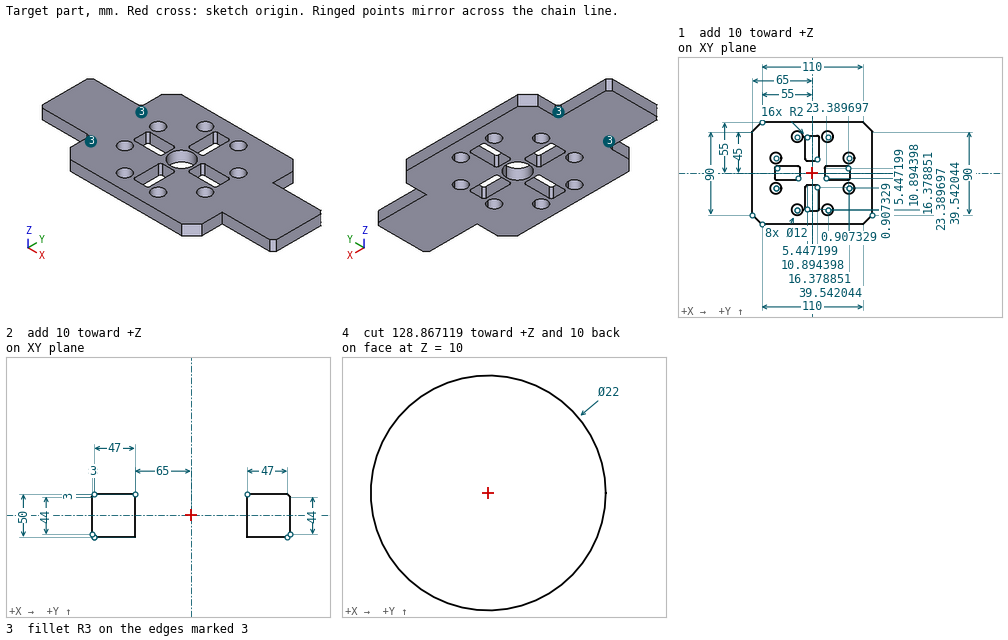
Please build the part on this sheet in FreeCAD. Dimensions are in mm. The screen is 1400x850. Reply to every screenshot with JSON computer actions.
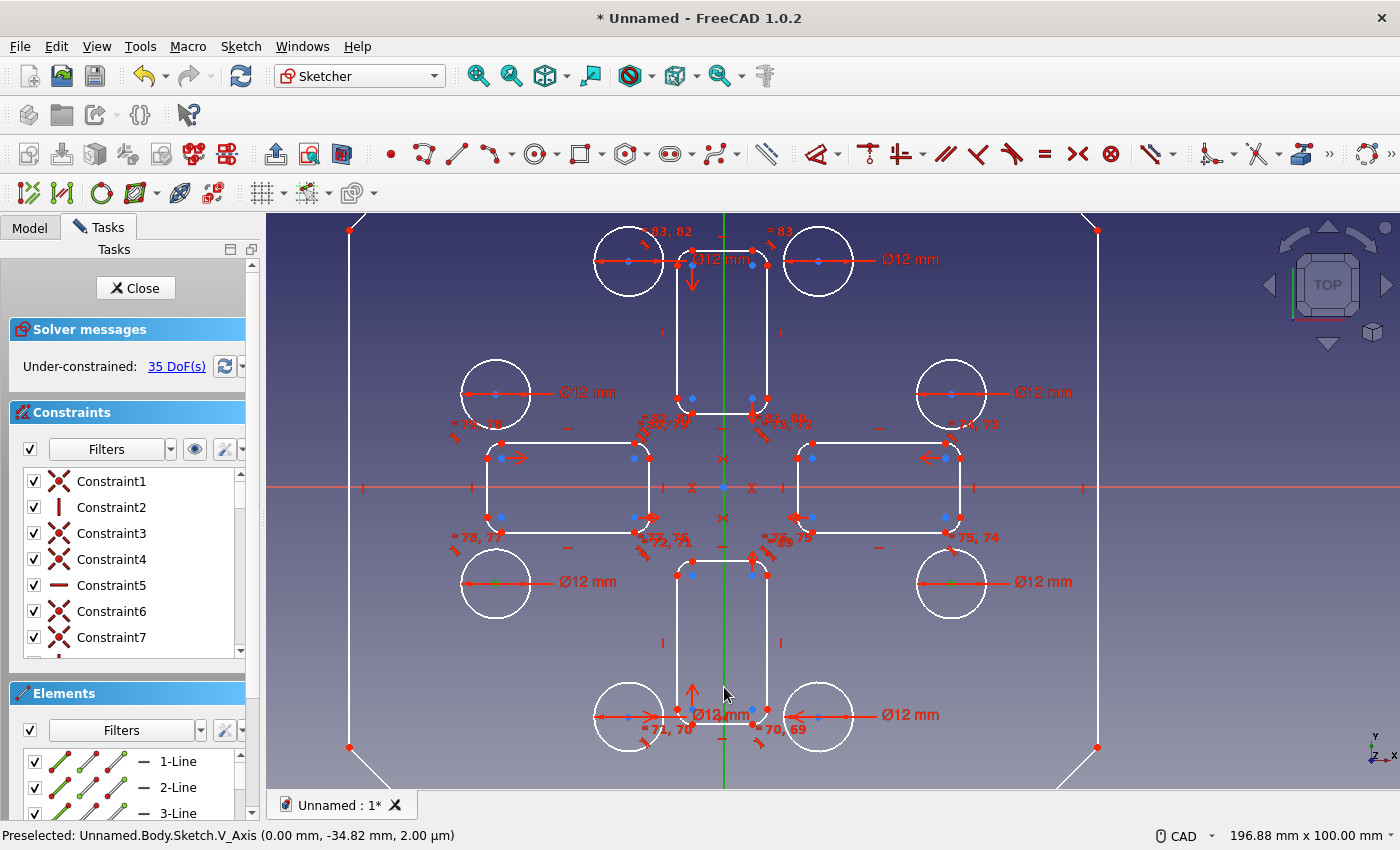
{"action": "left_click", "coordinate": [1078, 154]}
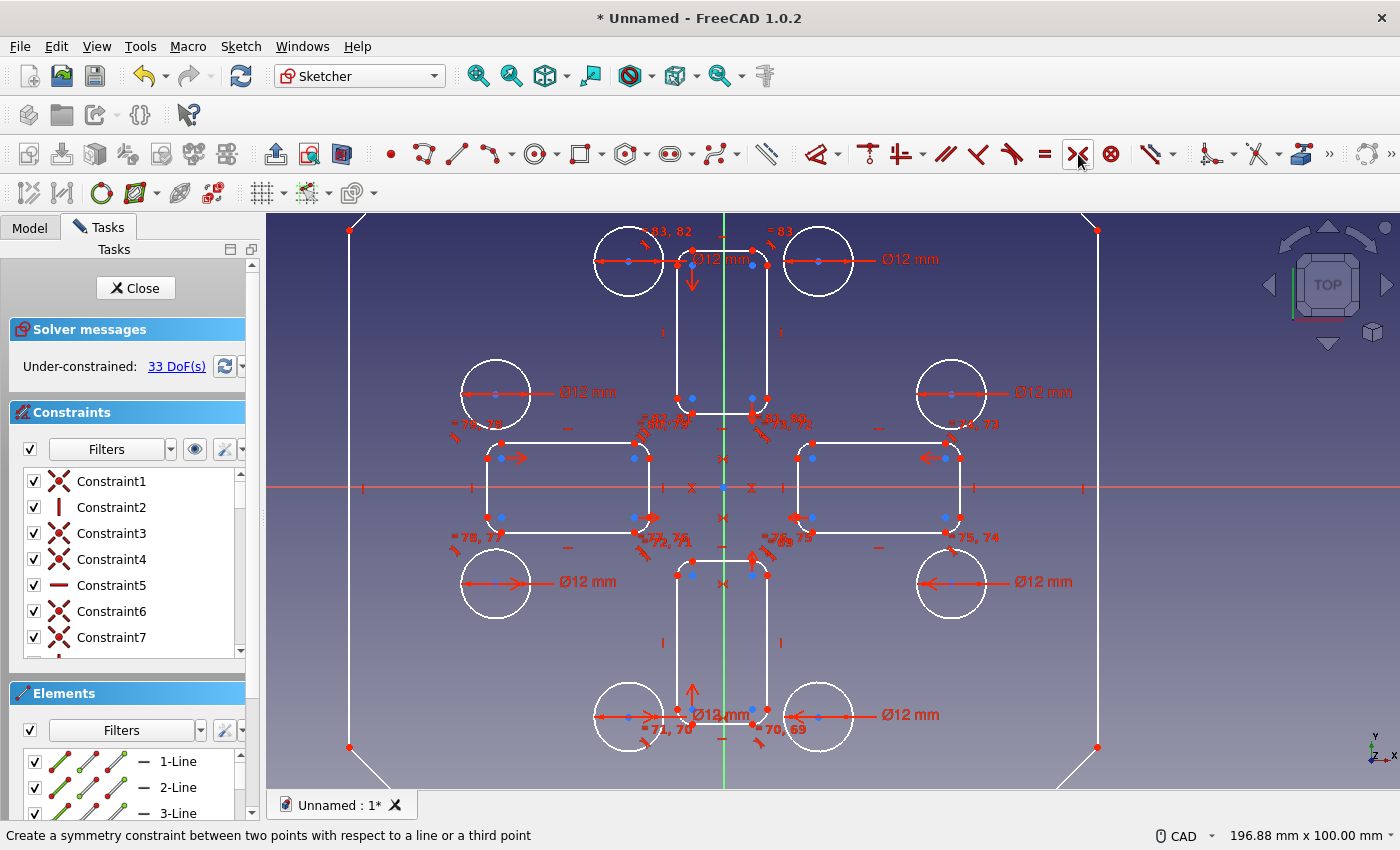
{"action": "left_click", "coordinate": [951, 584]}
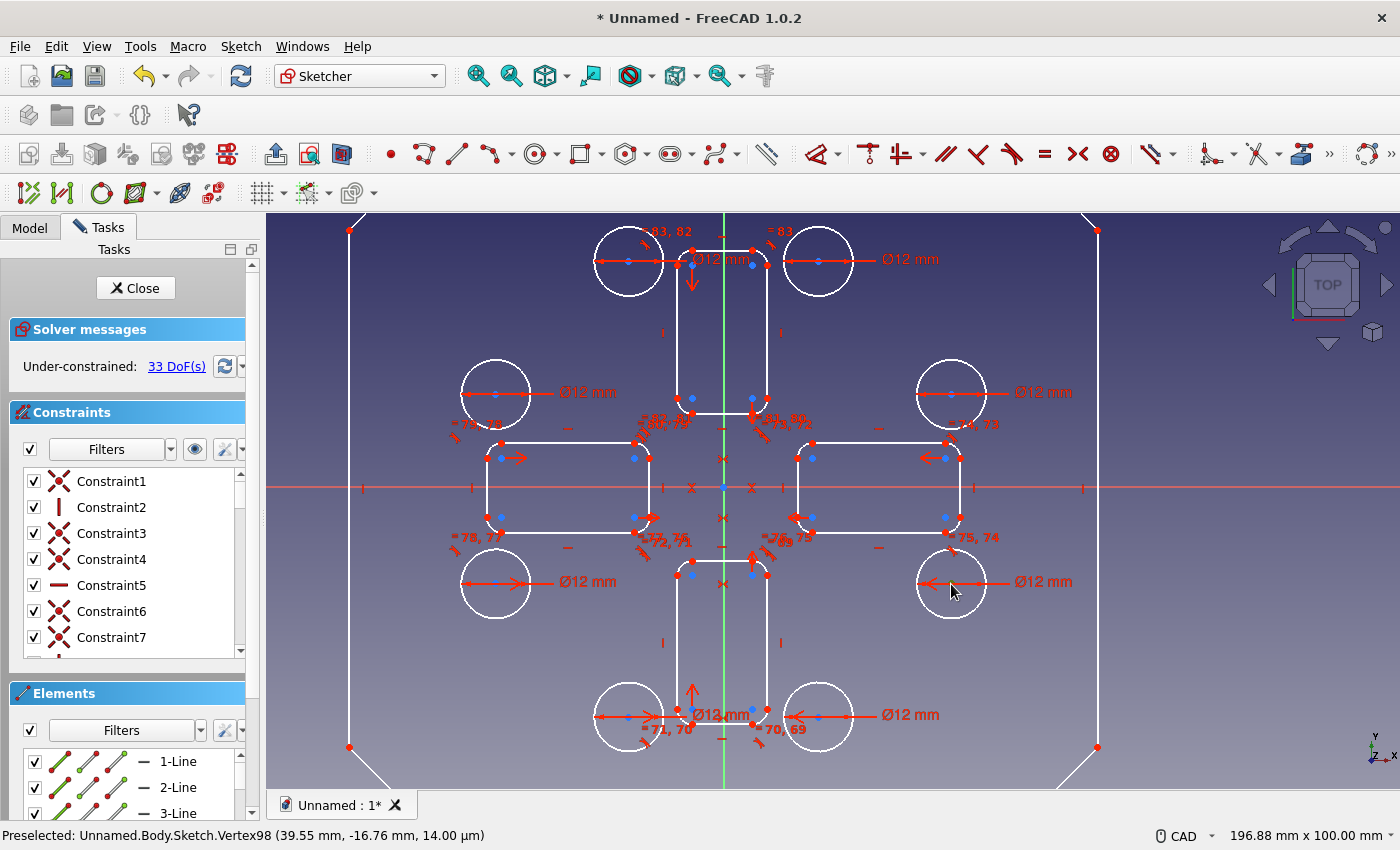
{"action": "left_click", "coordinate": [951, 394]}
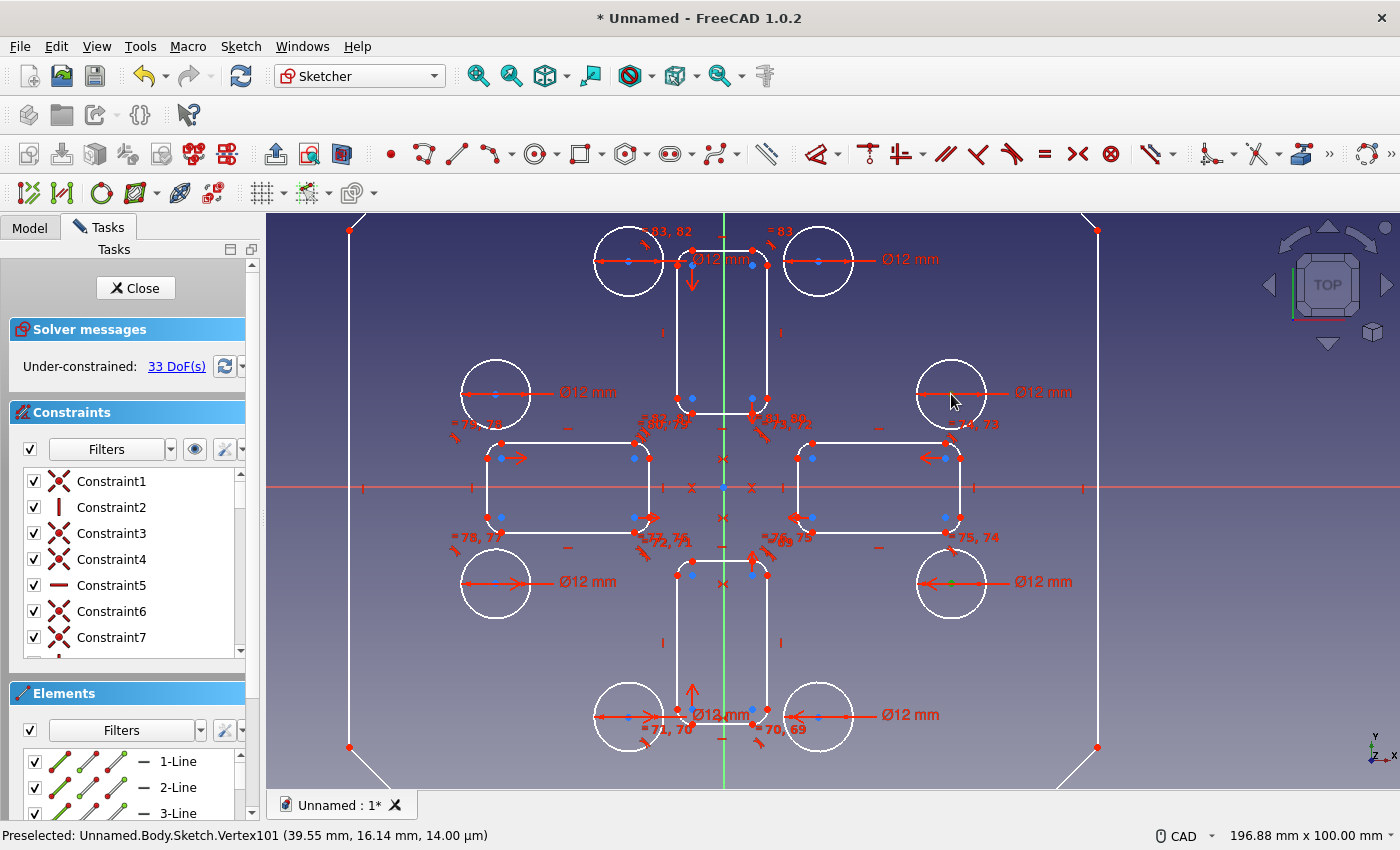
{"action": "left_click", "coordinate": [428, 487]}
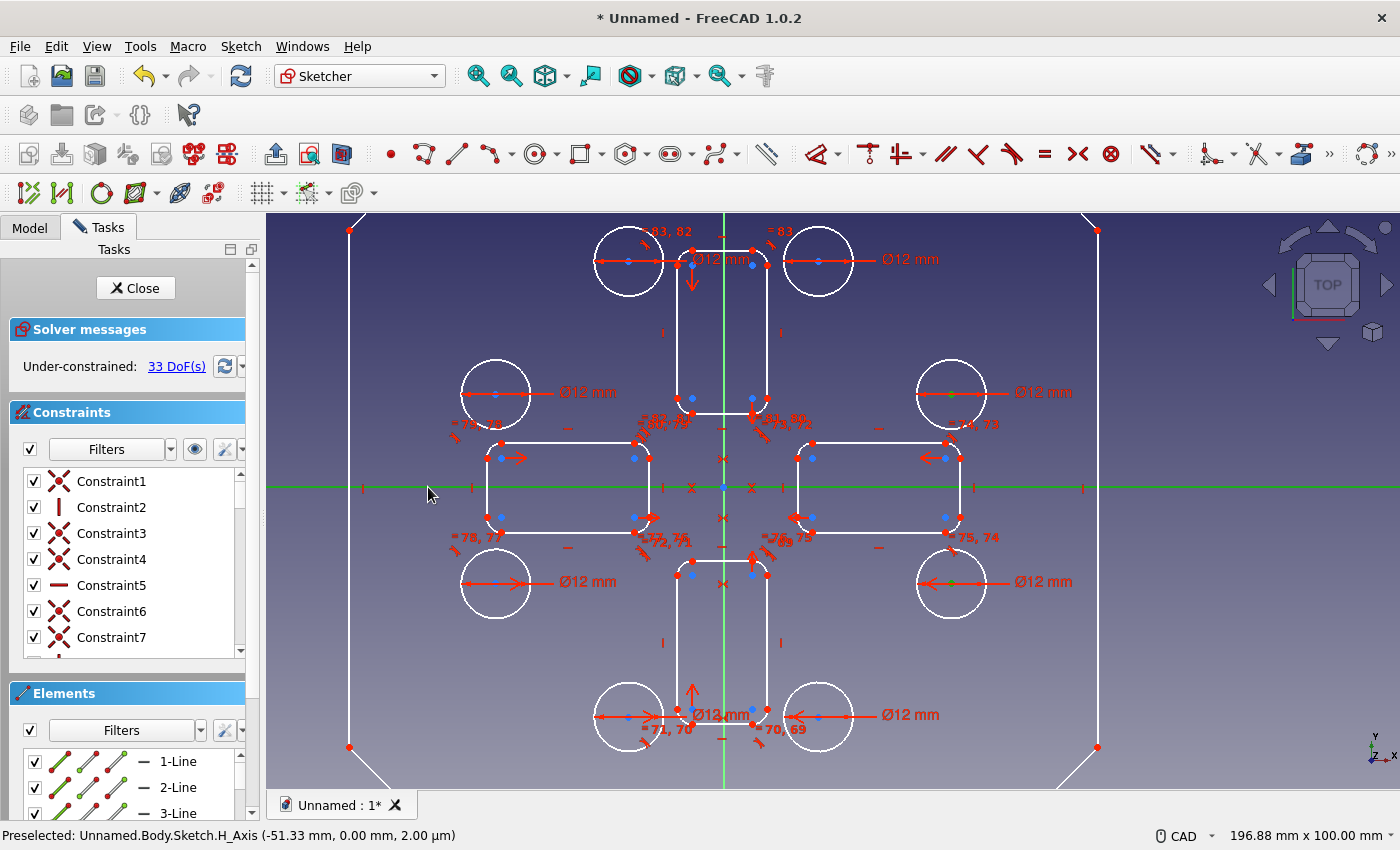
{"action": "left_click", "coordinate": [1078, 154]}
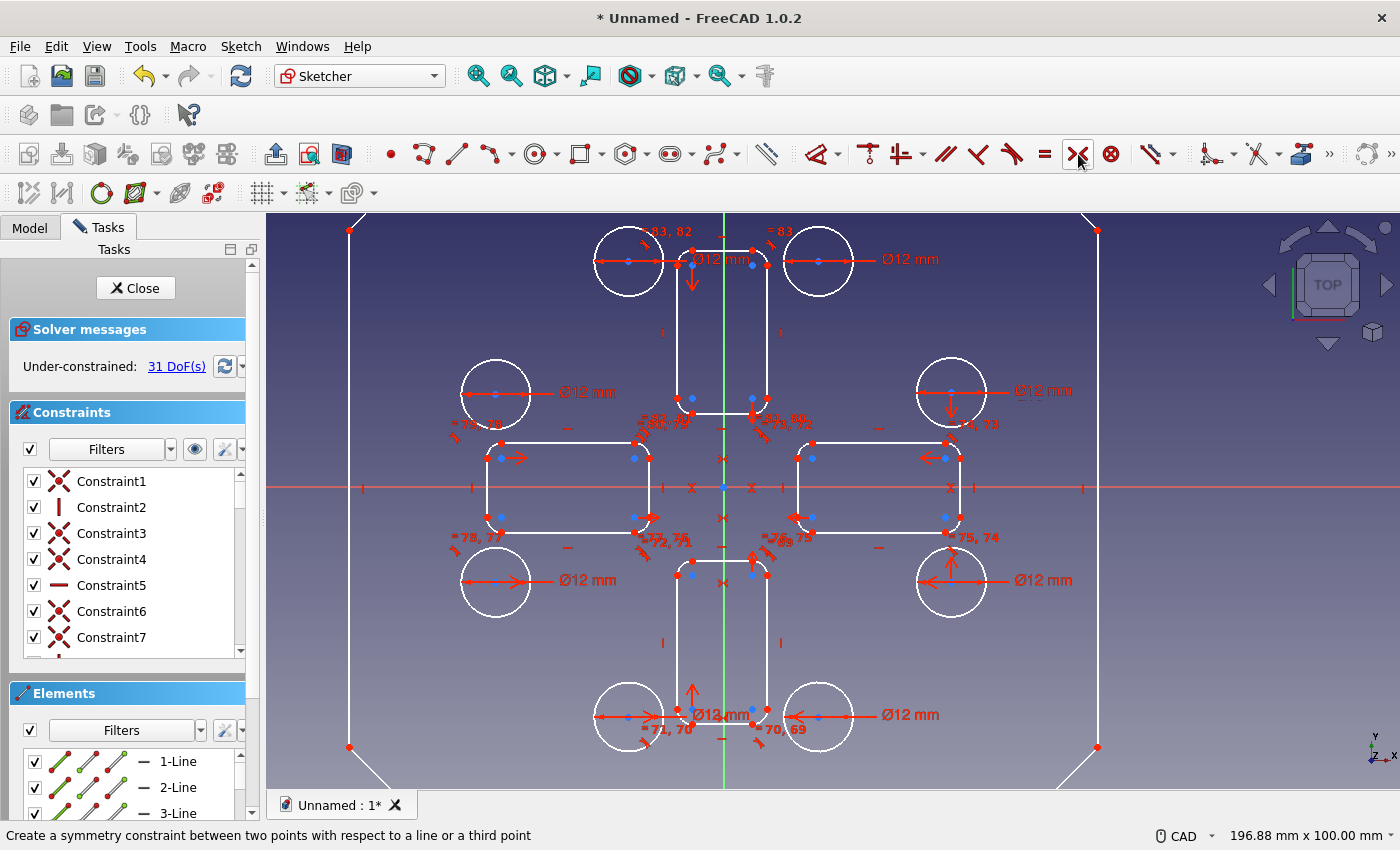
{"action": "left_click", "coordinate": [818, 717]}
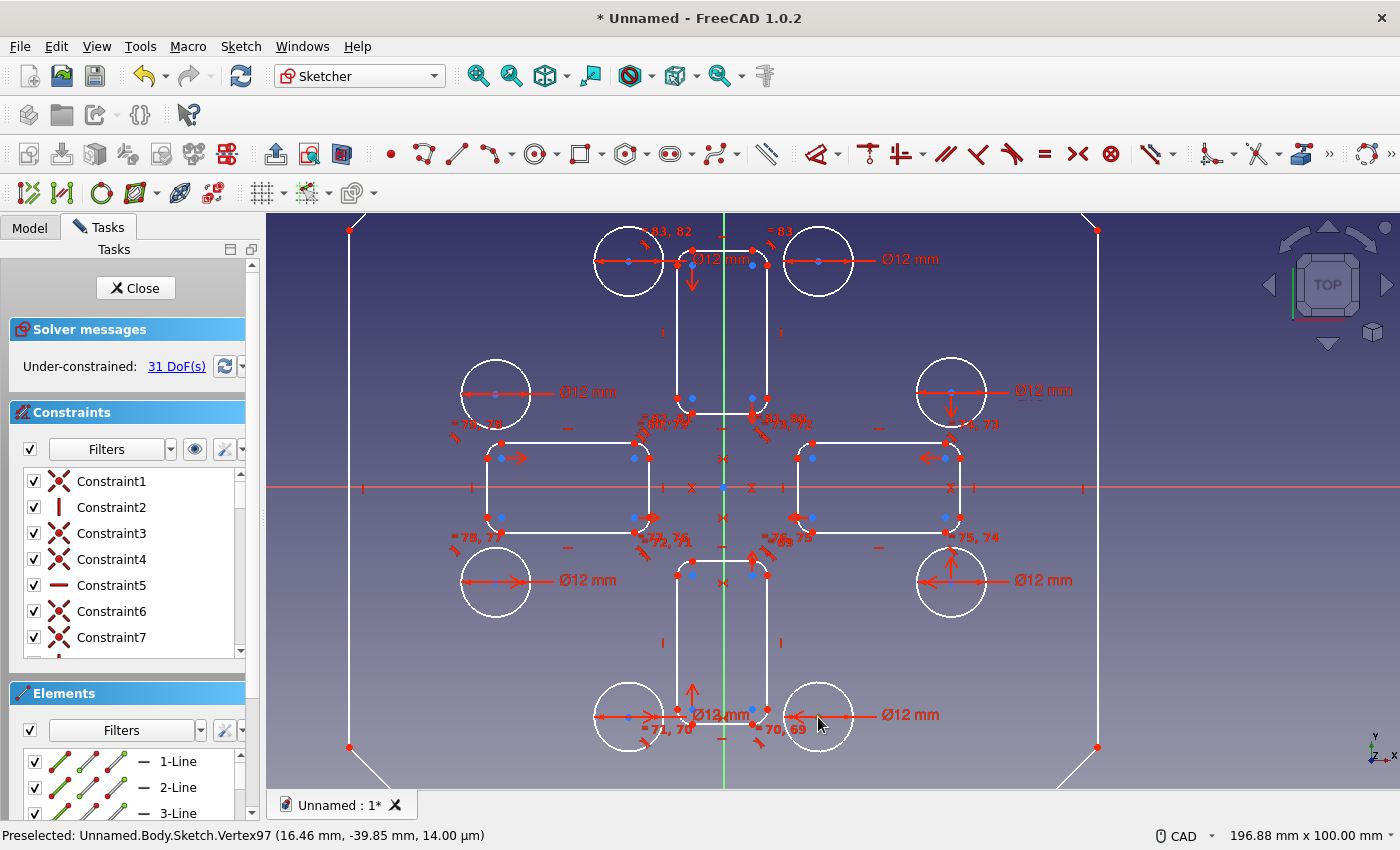
{"action": "left_click", "coordinate": [818, 261]}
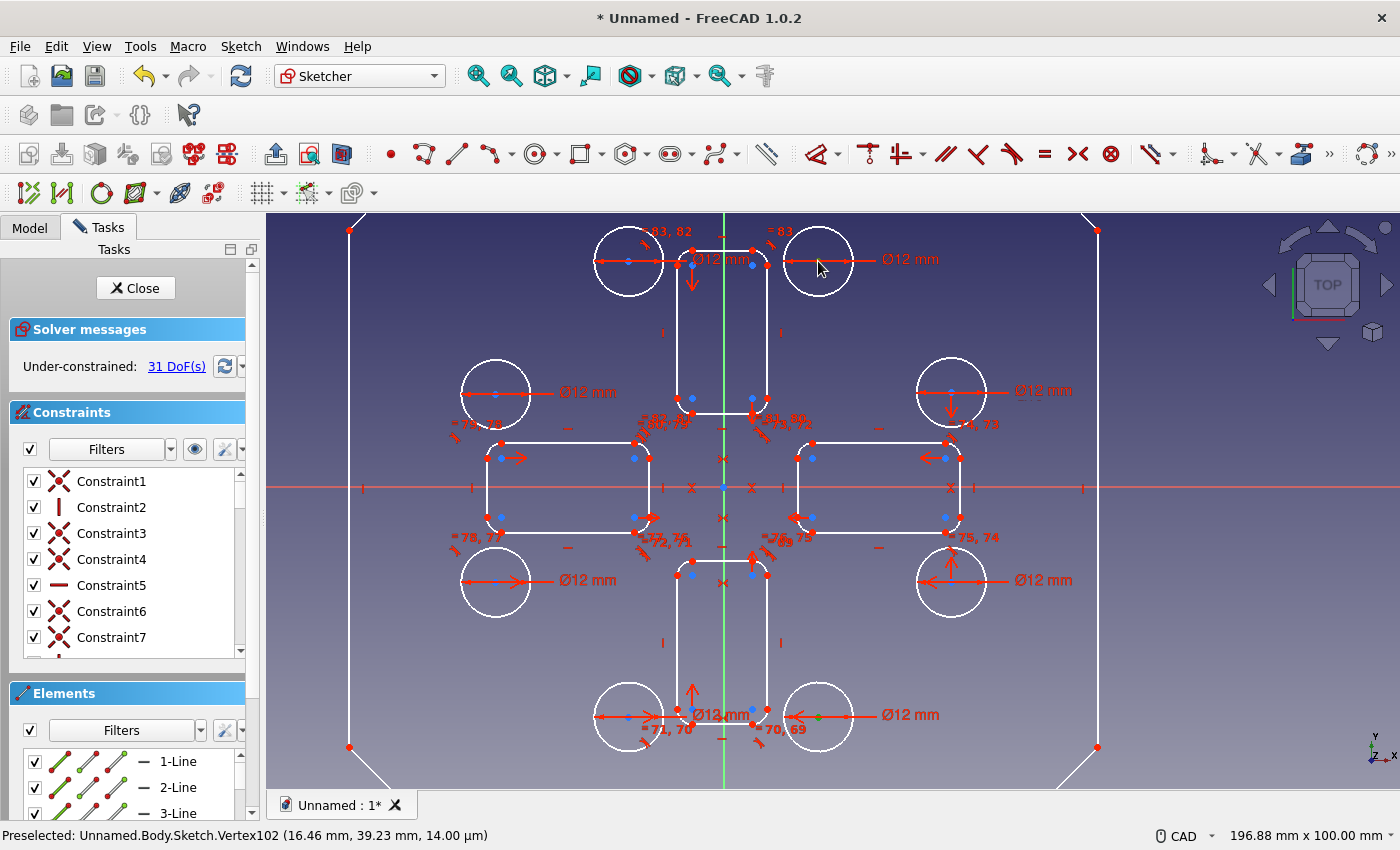
{"action": "left_click", "coordinate": [428, 487]}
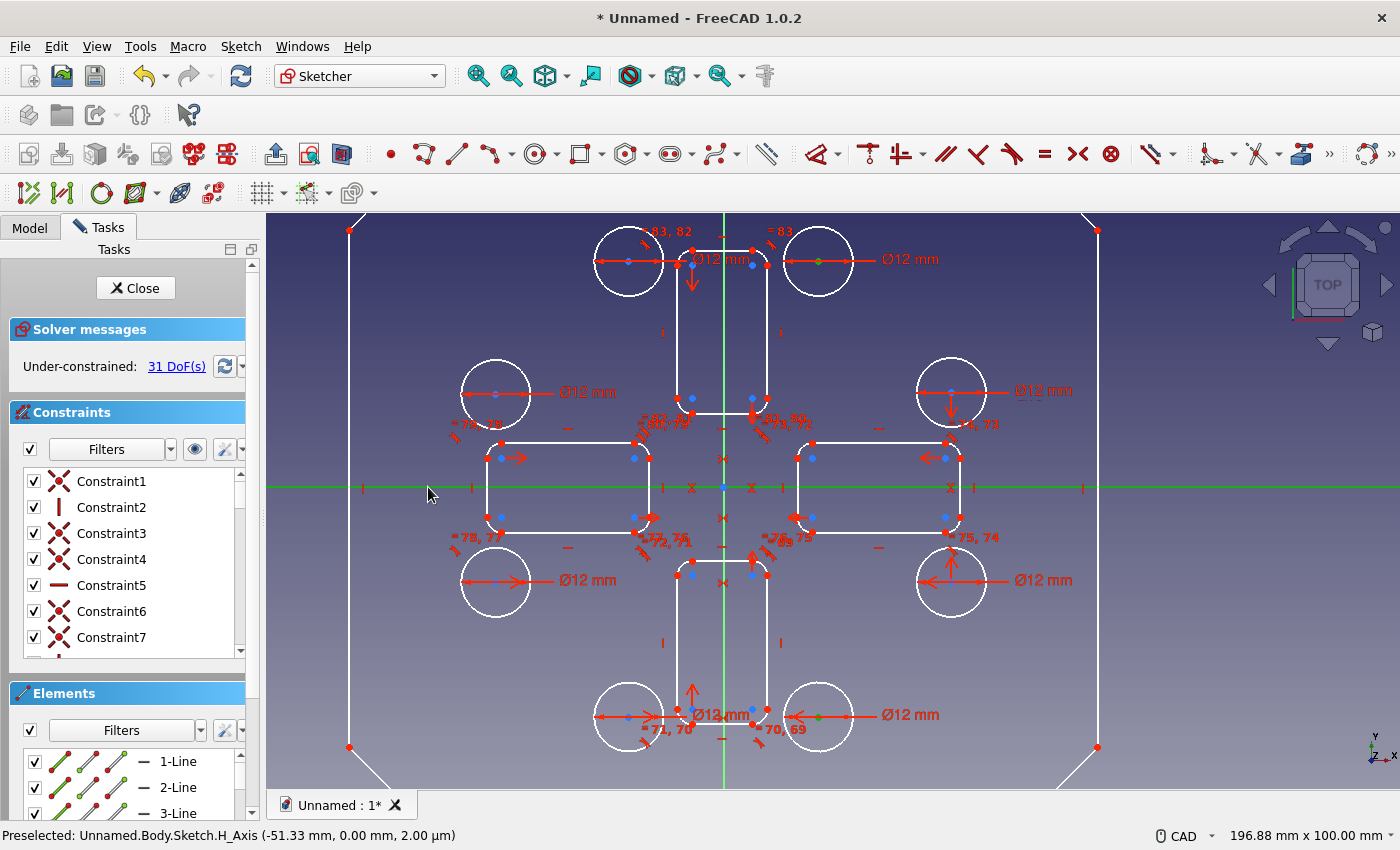
{"action": "left_click", "coordinate": [1078, 154]}